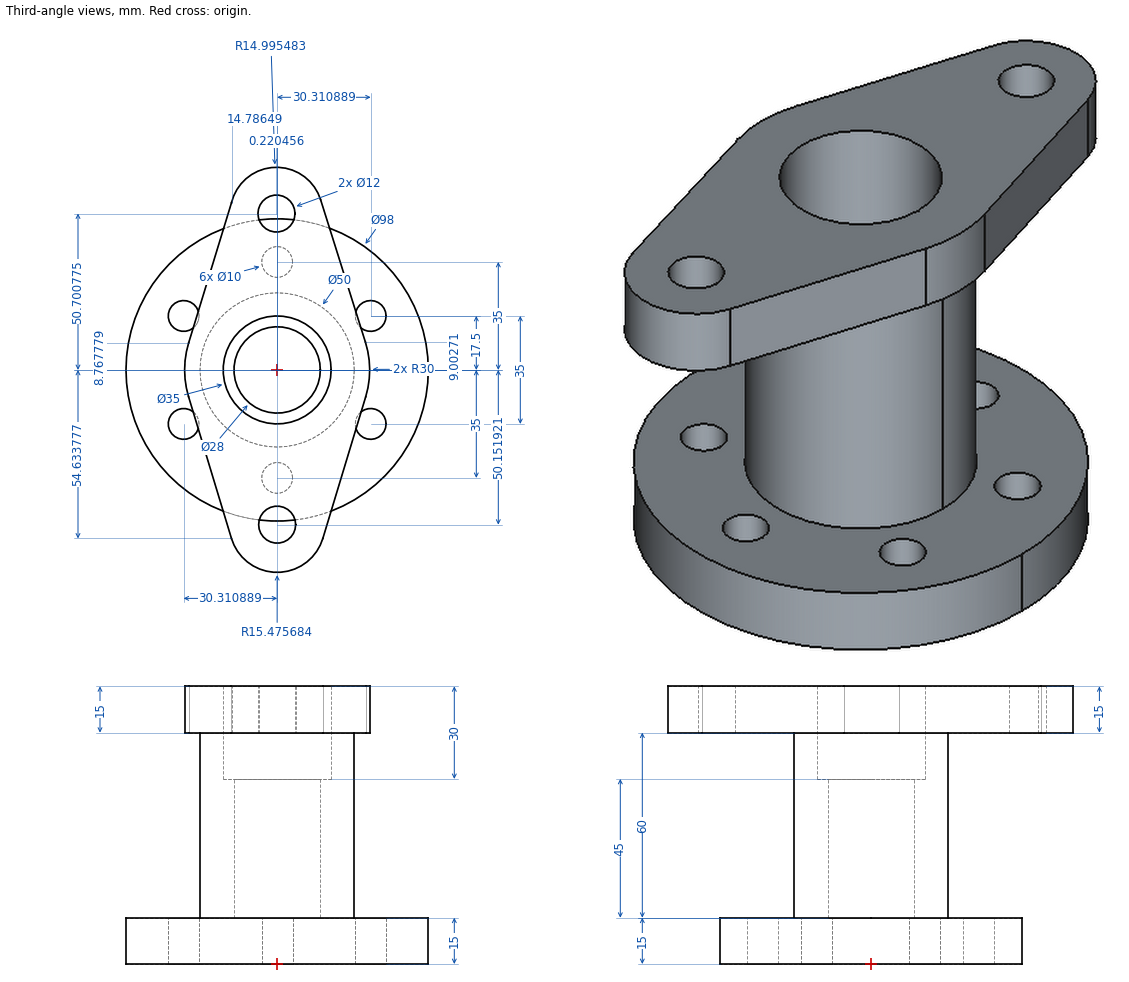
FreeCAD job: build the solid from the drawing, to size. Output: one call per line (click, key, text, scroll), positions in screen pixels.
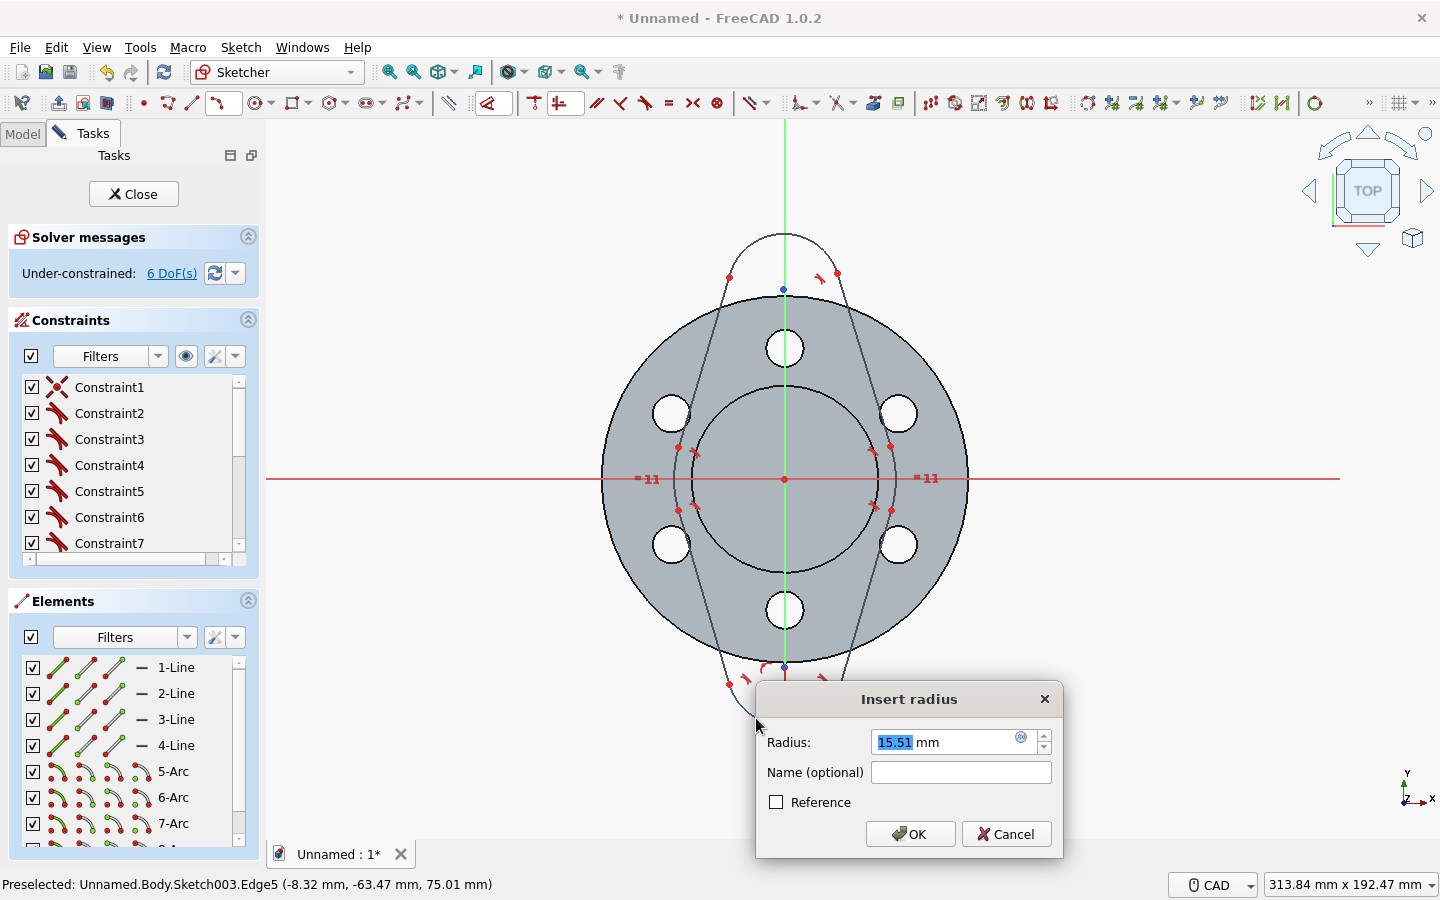
text(15.475684)
key(Return)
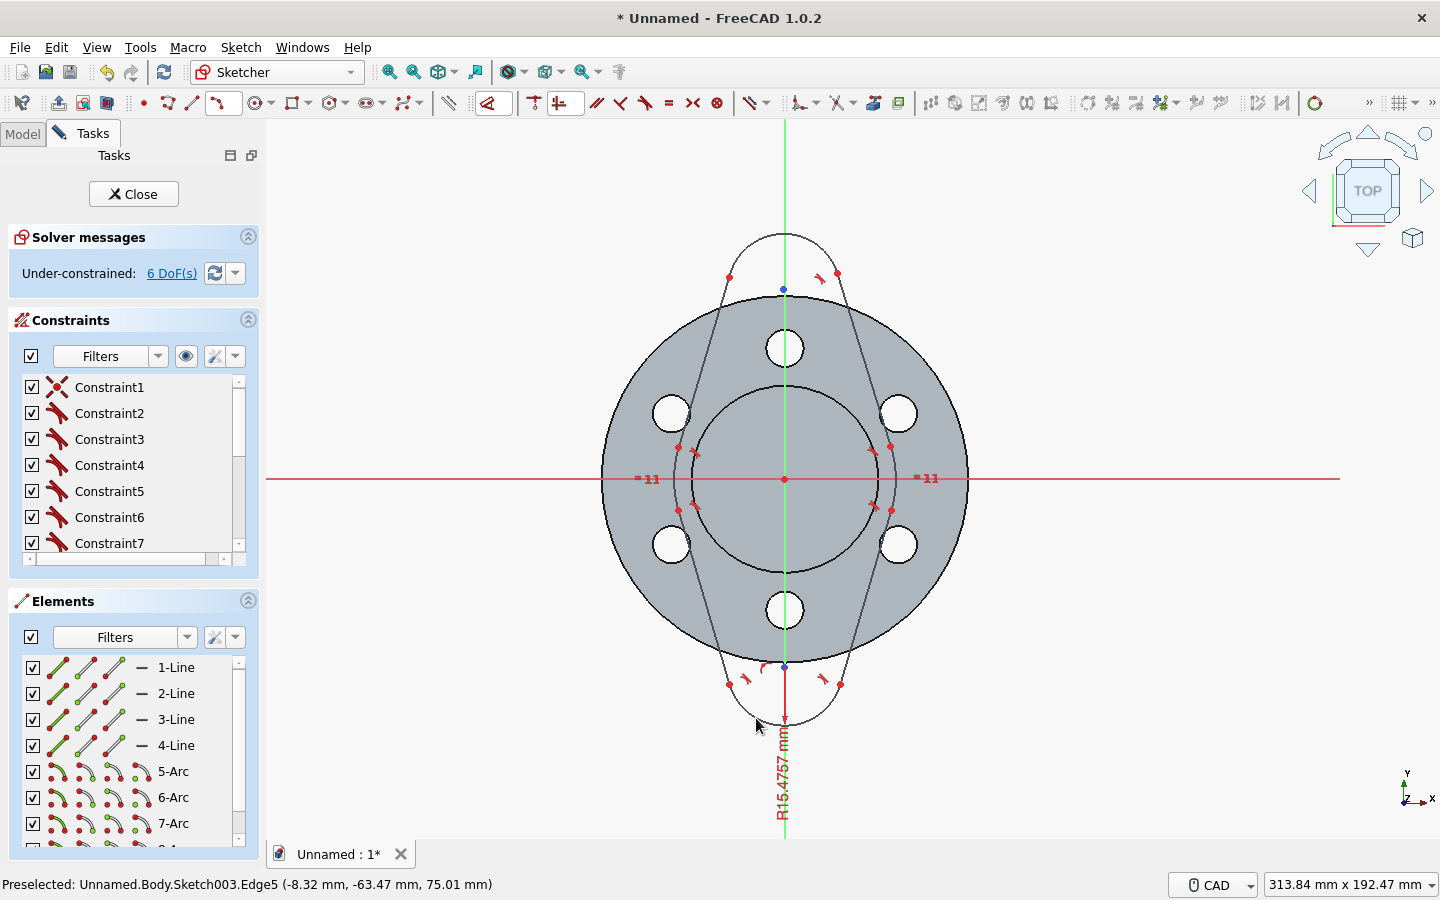
click(895, 491)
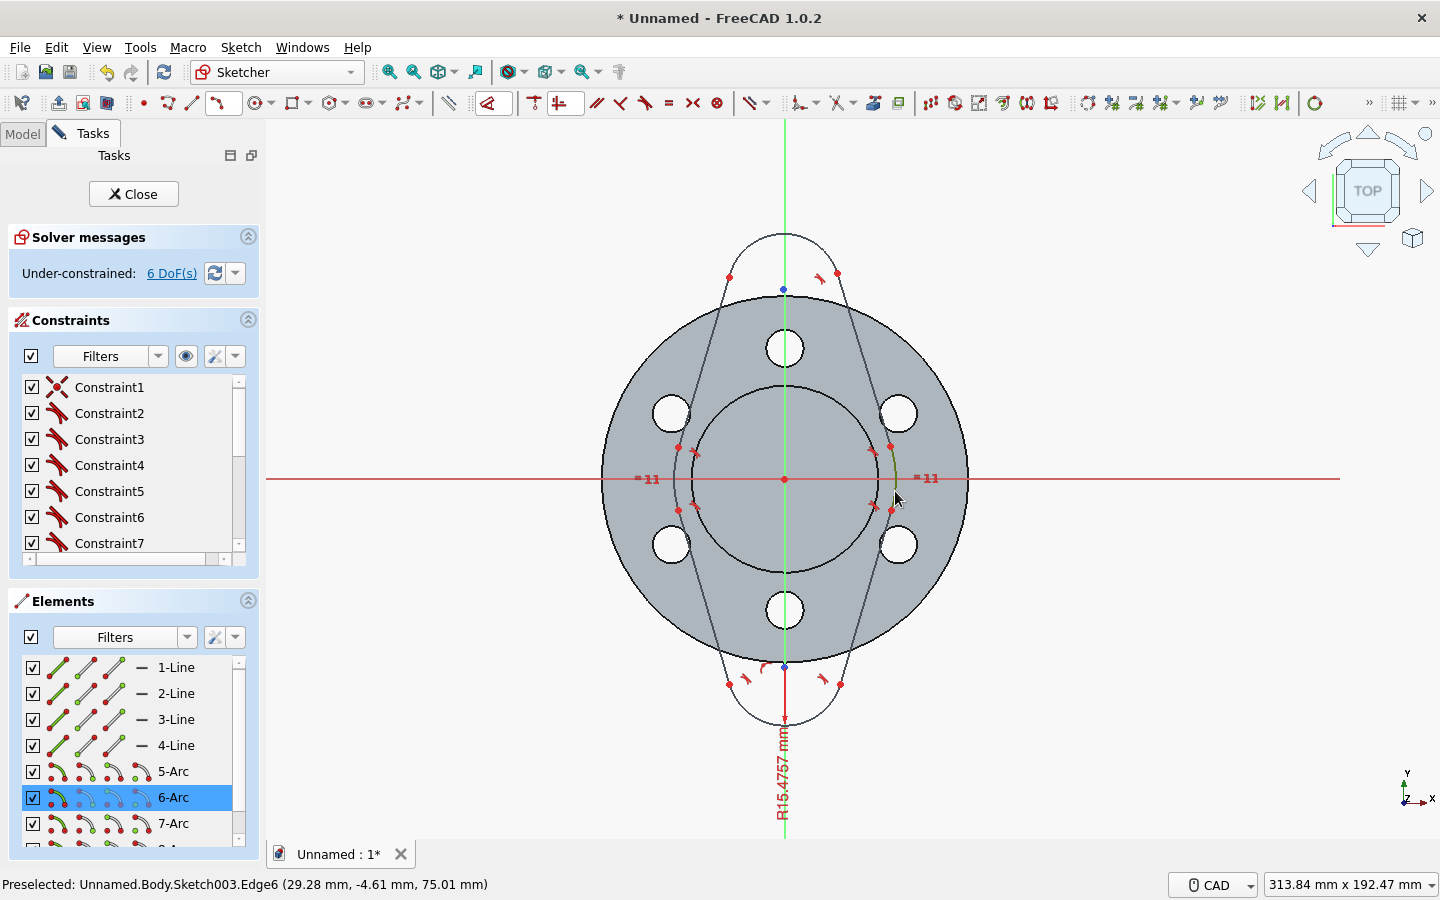
key(k)
key(r)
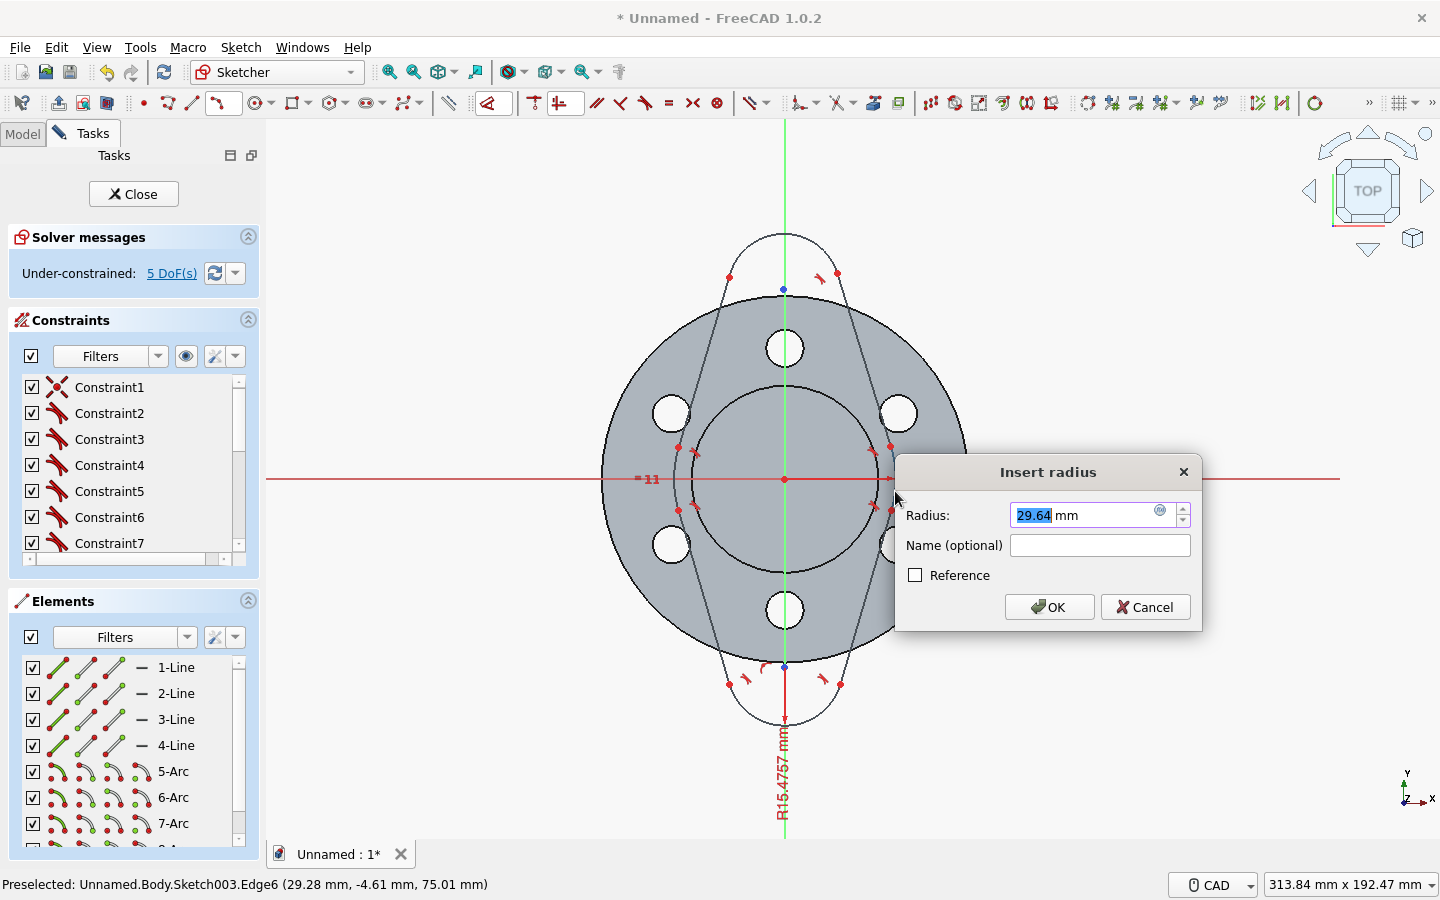
text(30)
key(Return)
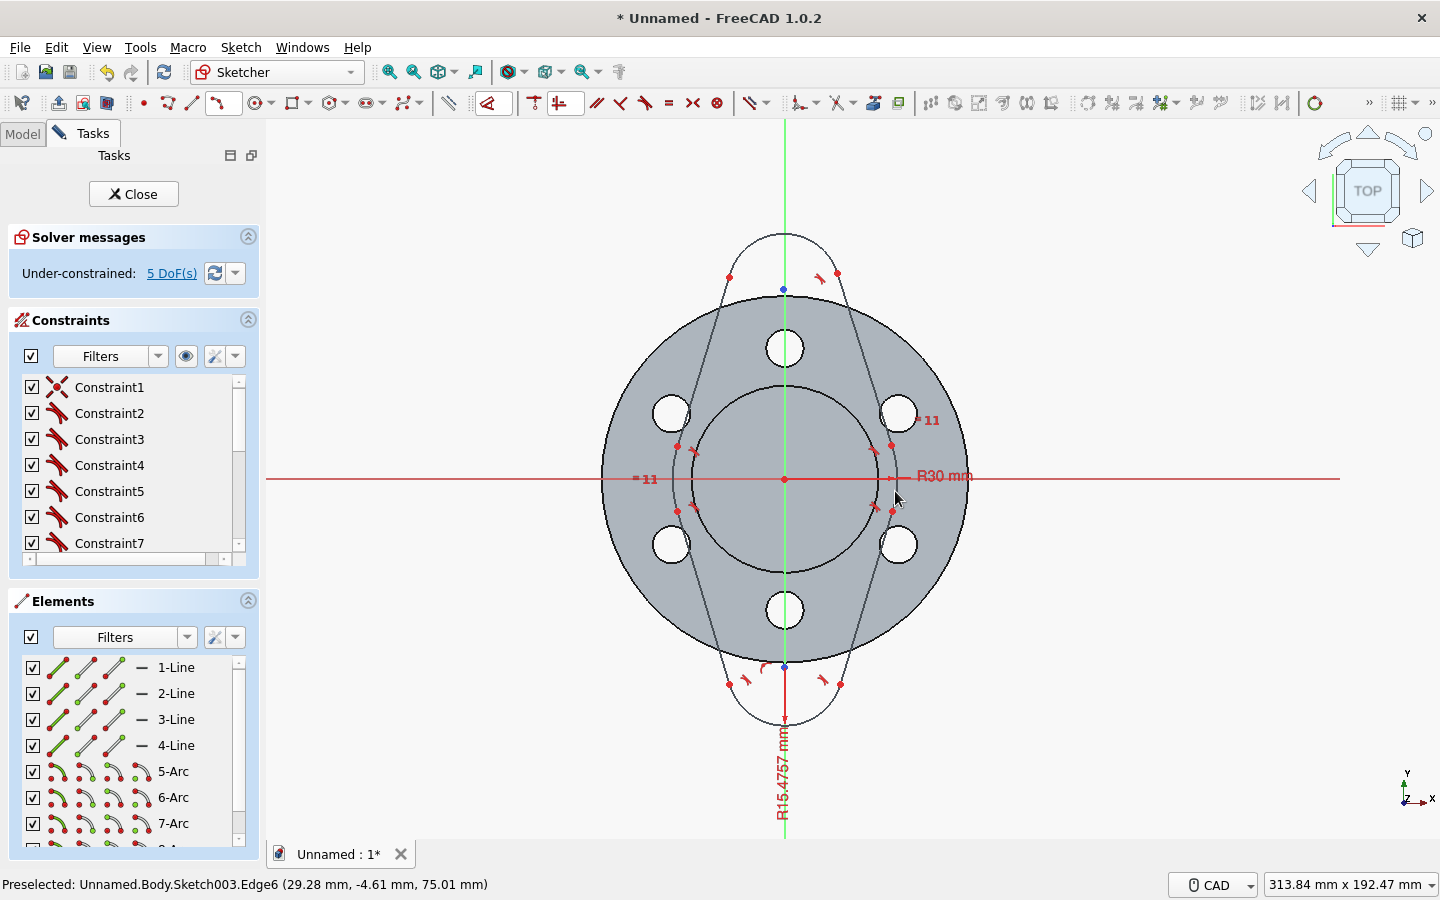
click(810, 240)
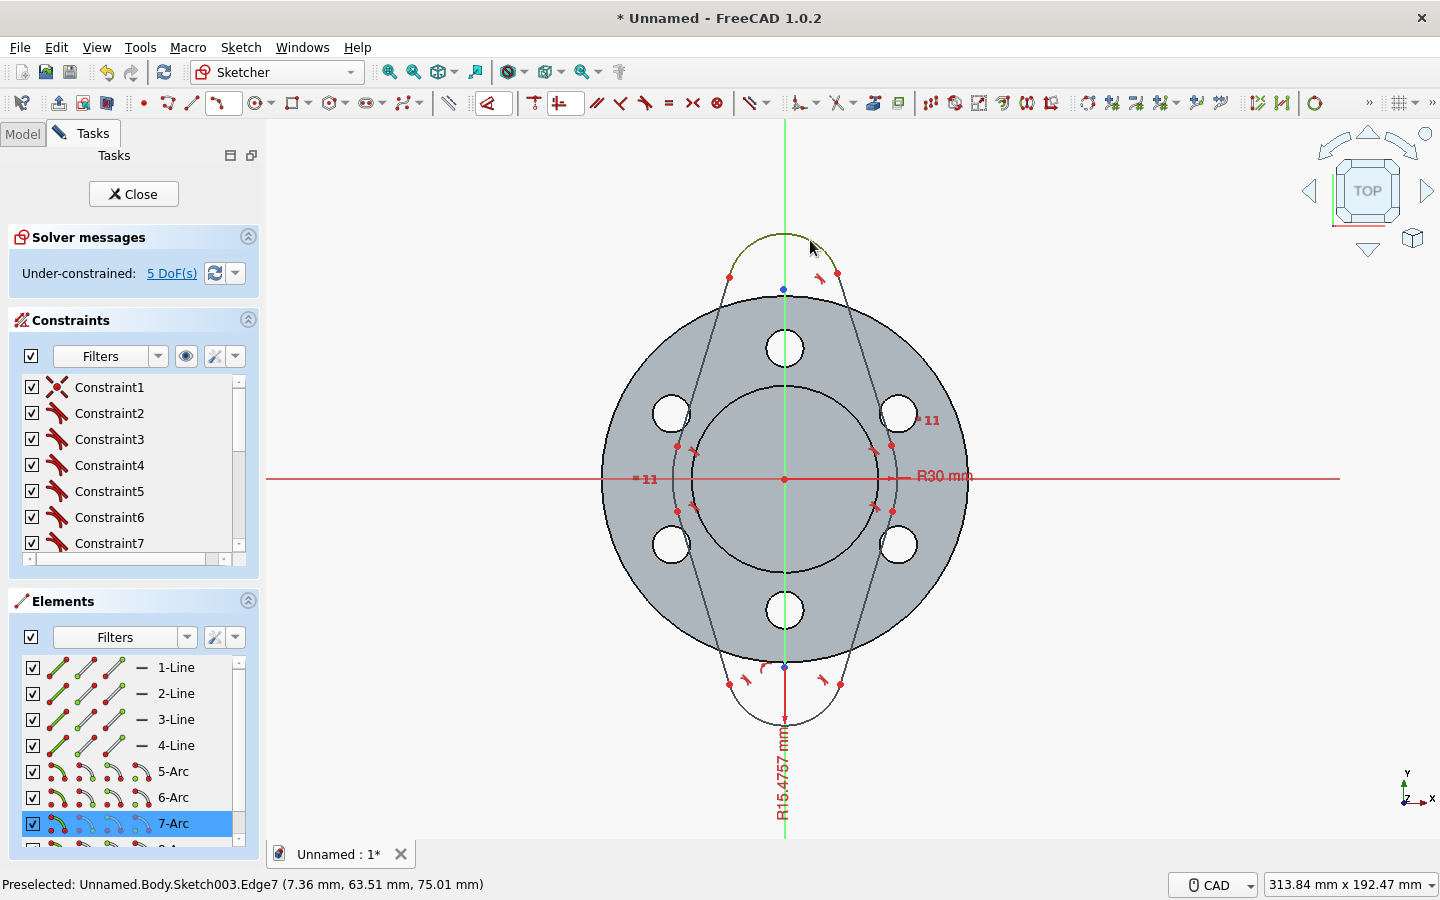
click(506, 104)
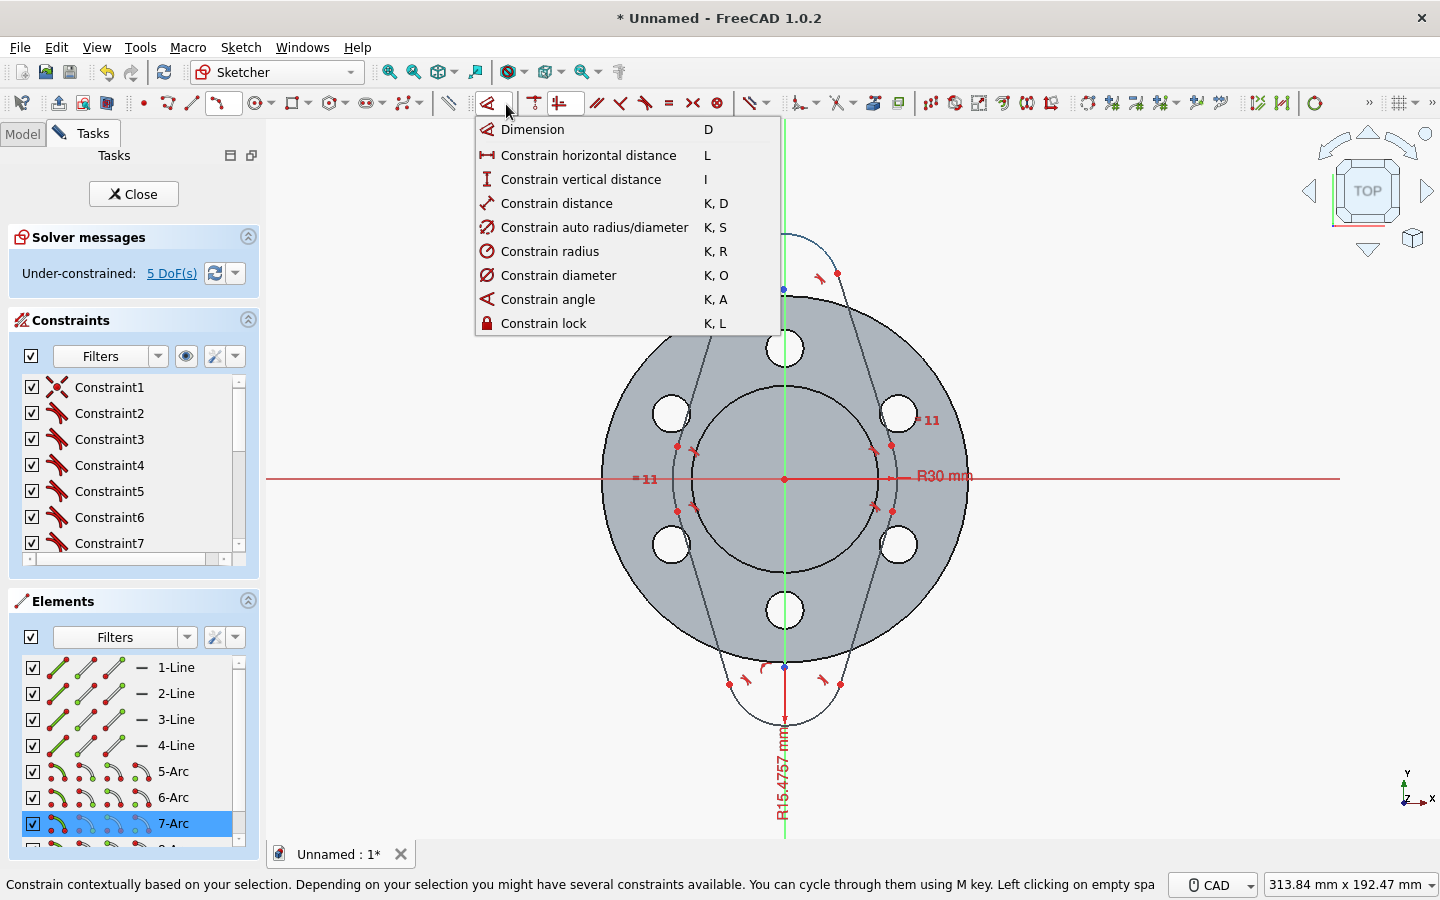
click(628, 251)